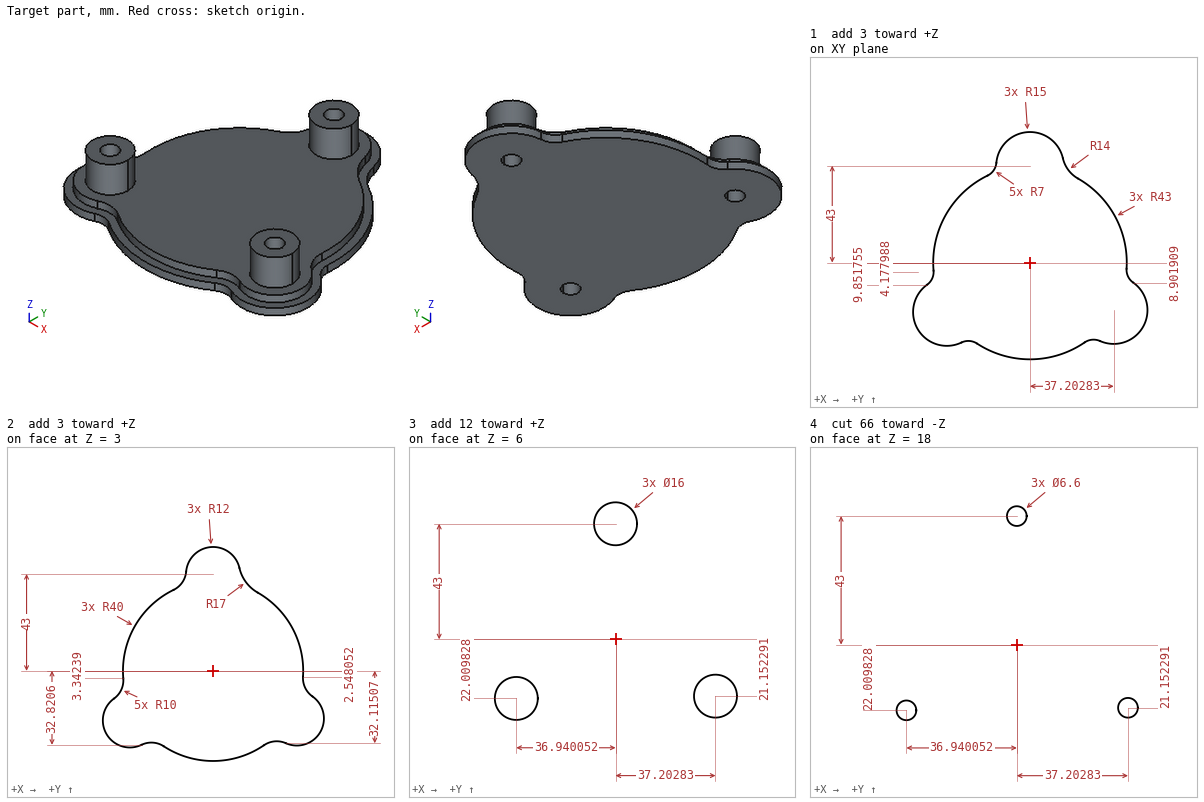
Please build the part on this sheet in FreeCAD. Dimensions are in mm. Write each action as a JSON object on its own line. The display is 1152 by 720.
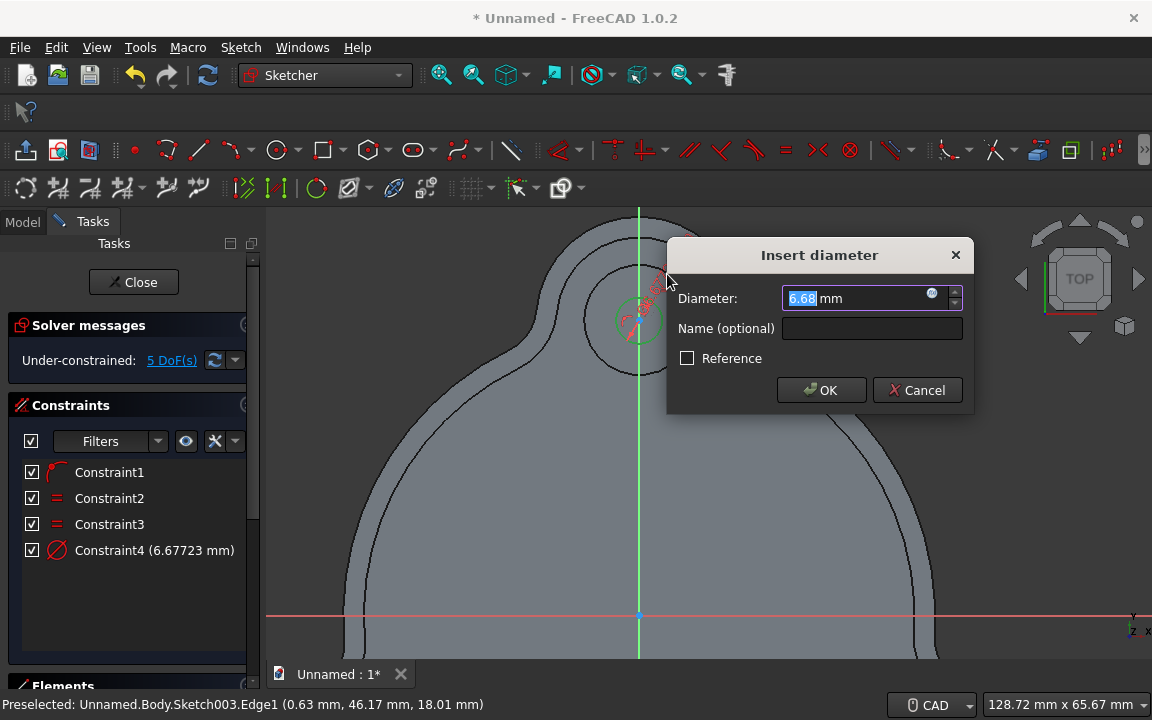
{"action": "type", "text": "6.6"}
{"action": "key", "text": "Return"}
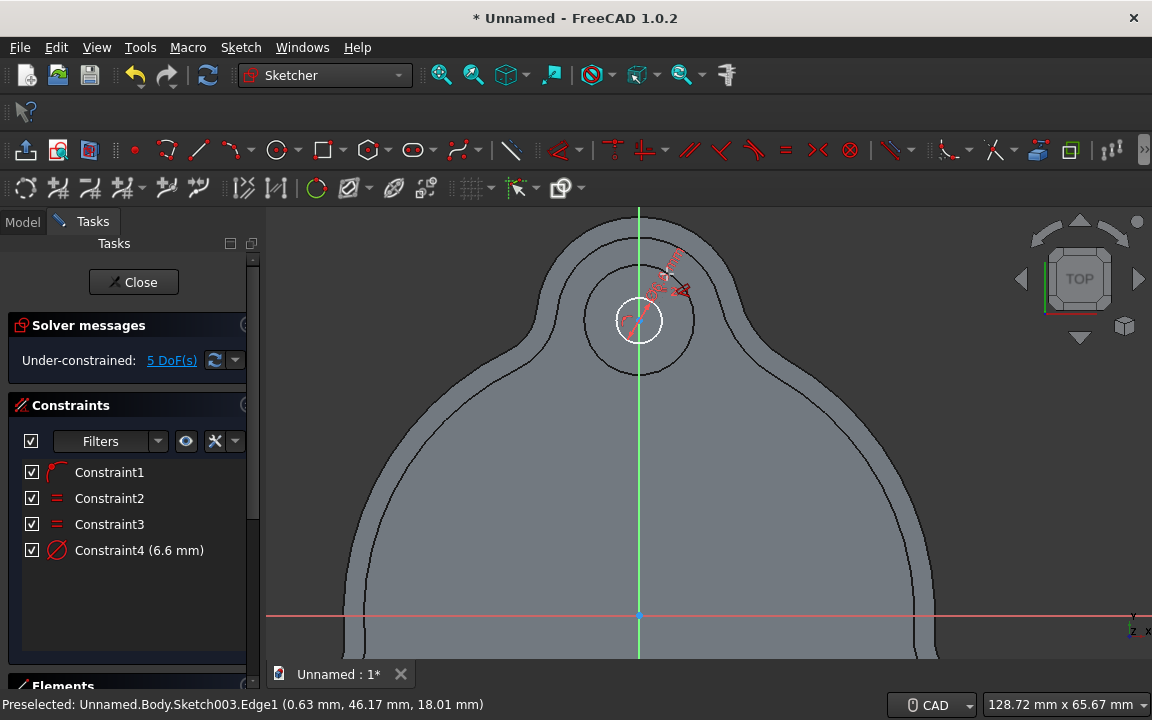
{"action": "left_click", "coordinate": [639, 321]}
{"action": "left_click", "coordinate": [605, 468]}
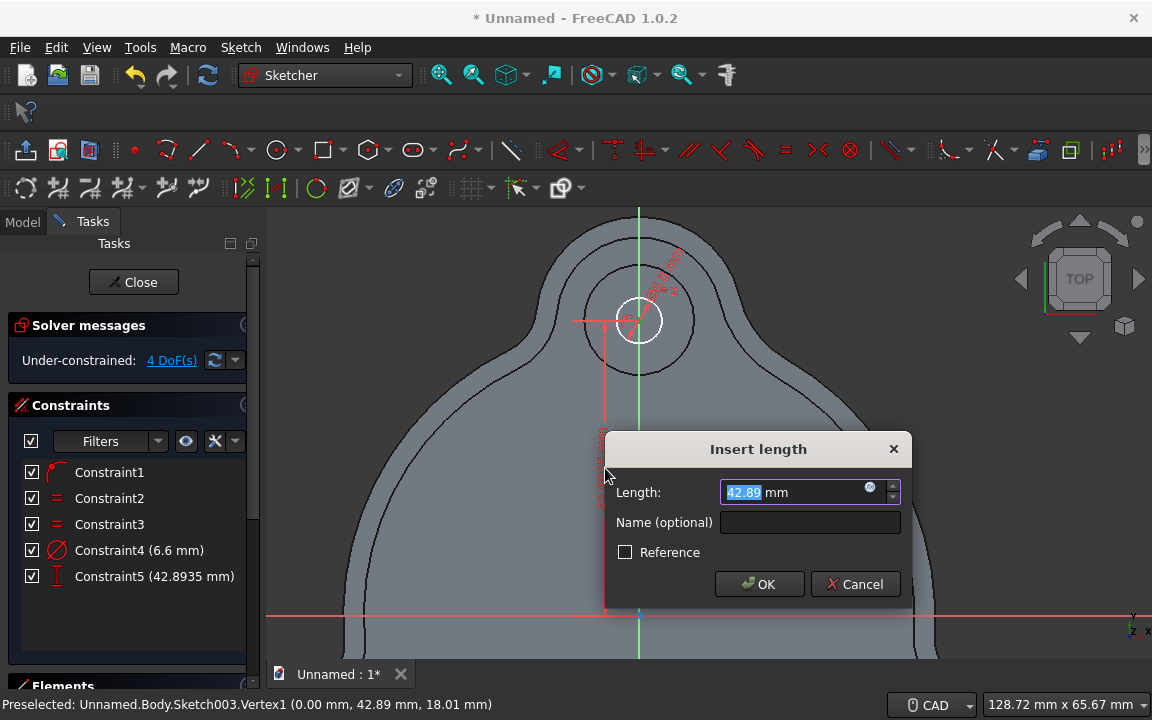
{"action": "type", "text": "43"}
{"action": "key", "text": "Return"}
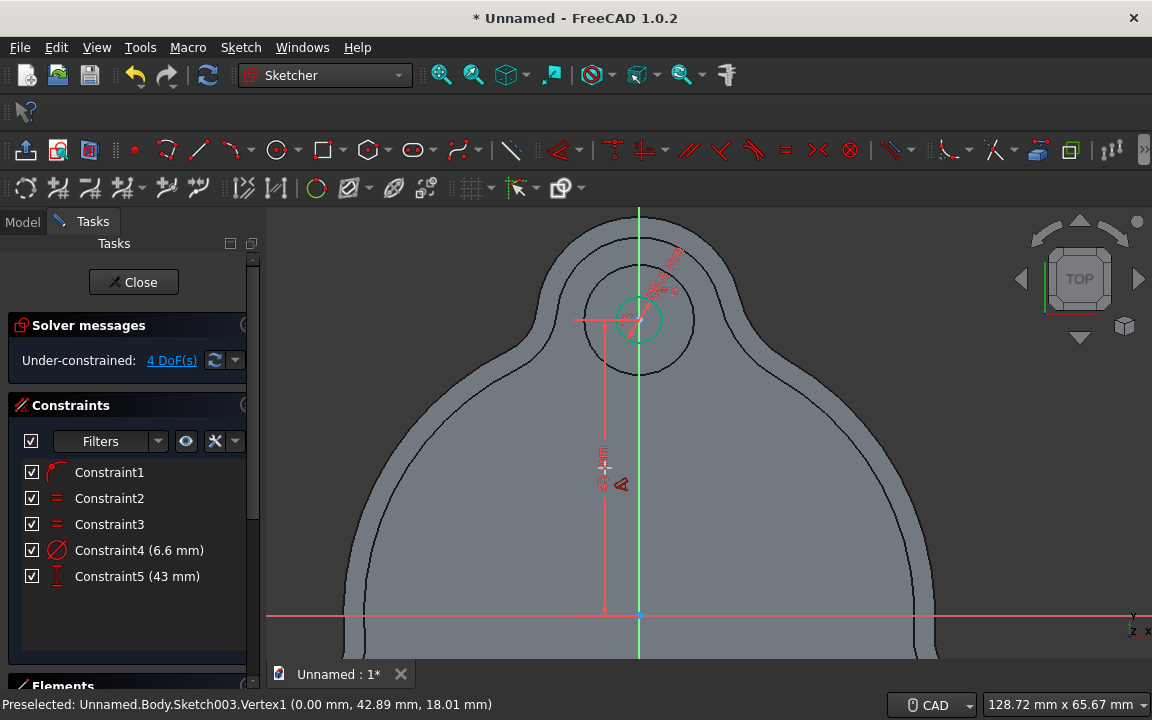
{"action": "scroll", "coordinate": [641, 298], "scroll_direction": "down", "scroll_amount": 3}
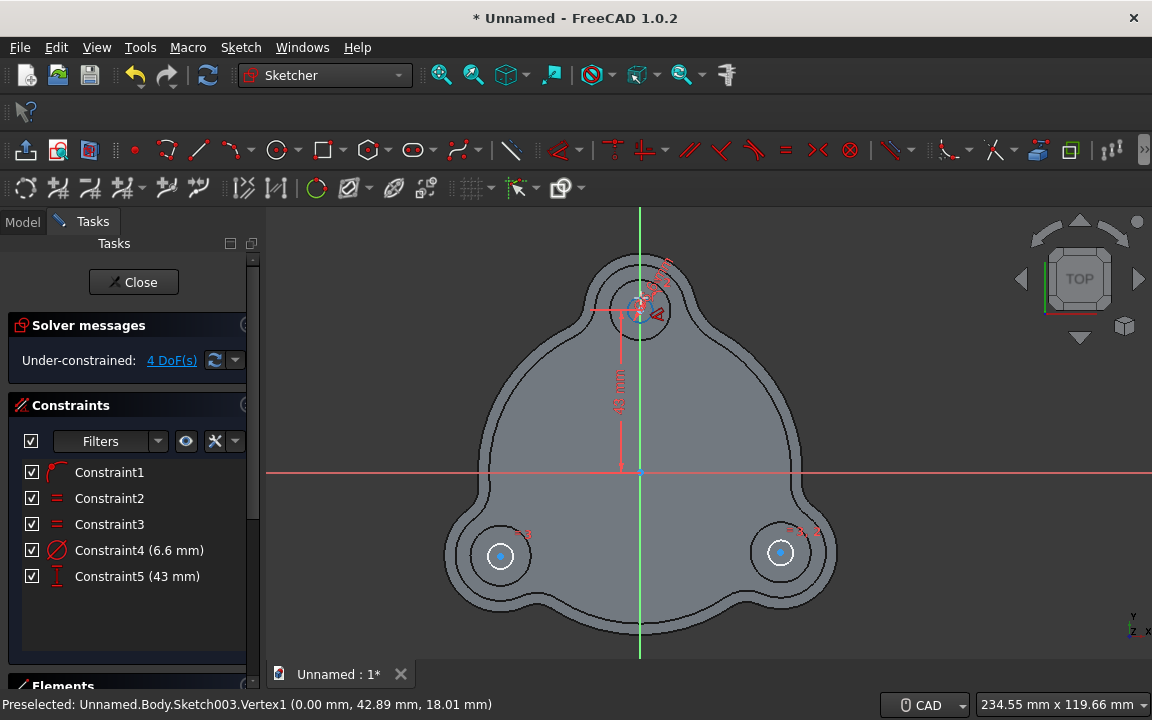
{"action": "left_click", "coordinate": [781, 553]}
{"action": "left_click", "coordinate": [710, 587]}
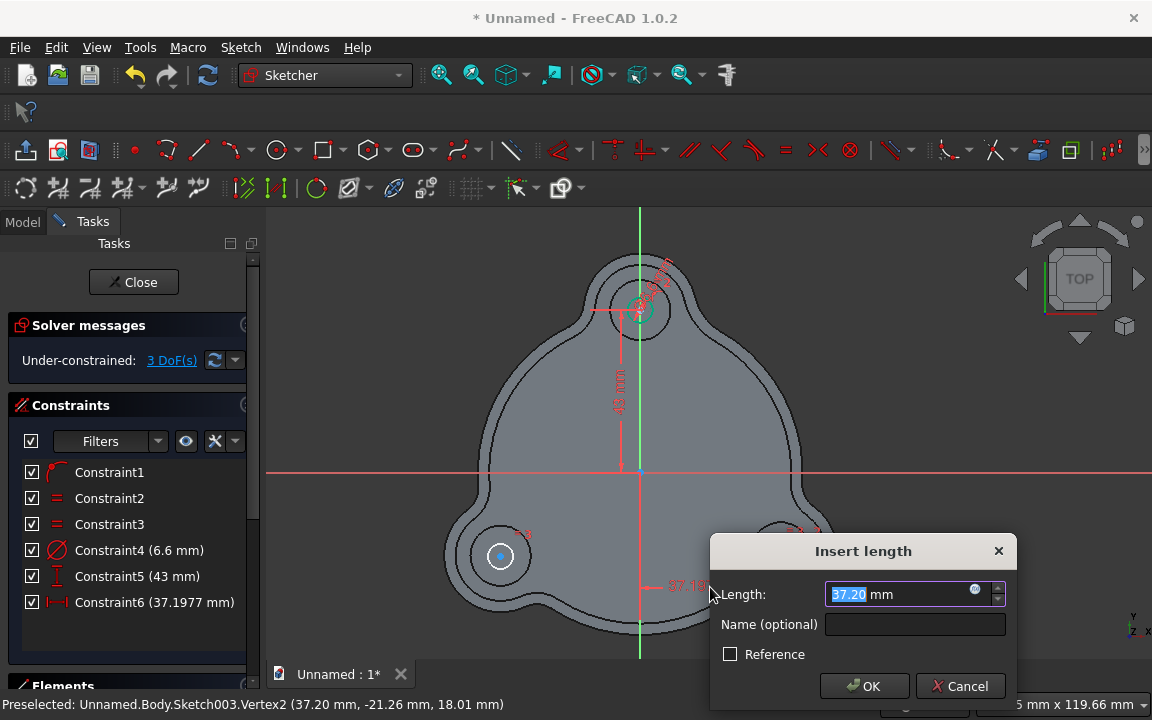
{"action": "type", "text": "37.20283"}
{"action": "key", "text": "Return"}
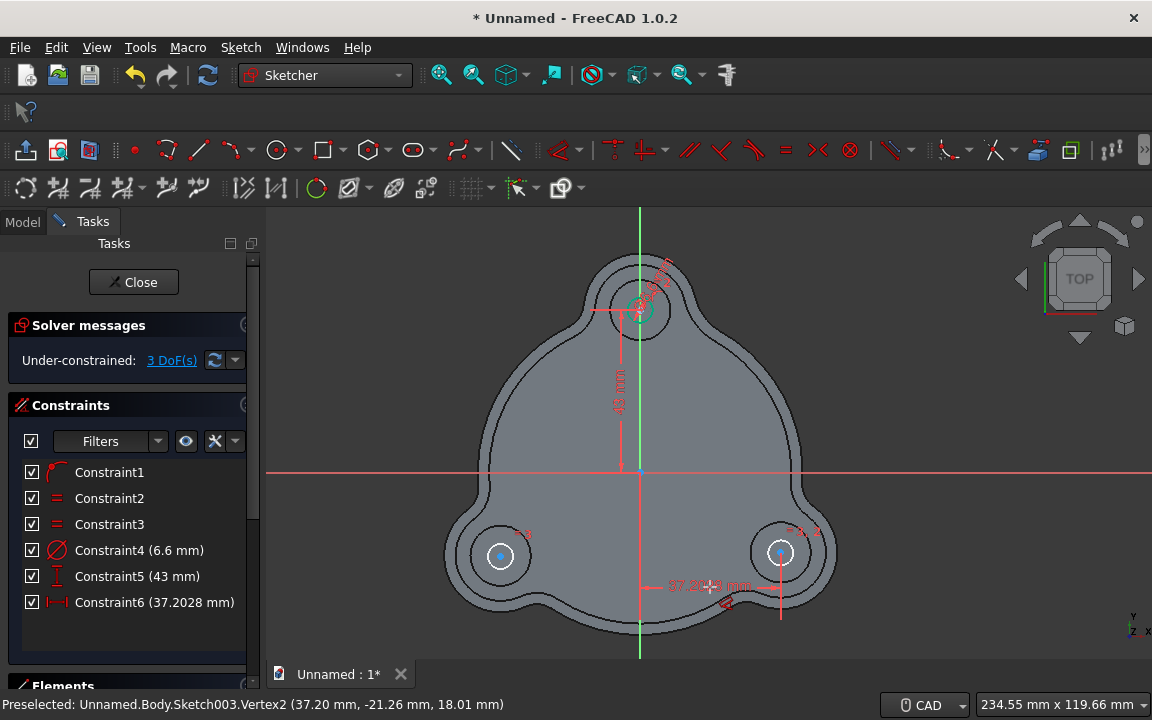
{"action": "left_click", "coordinate": [781, 553]}
{"action": "left_click", "coordinate": [815, 513]}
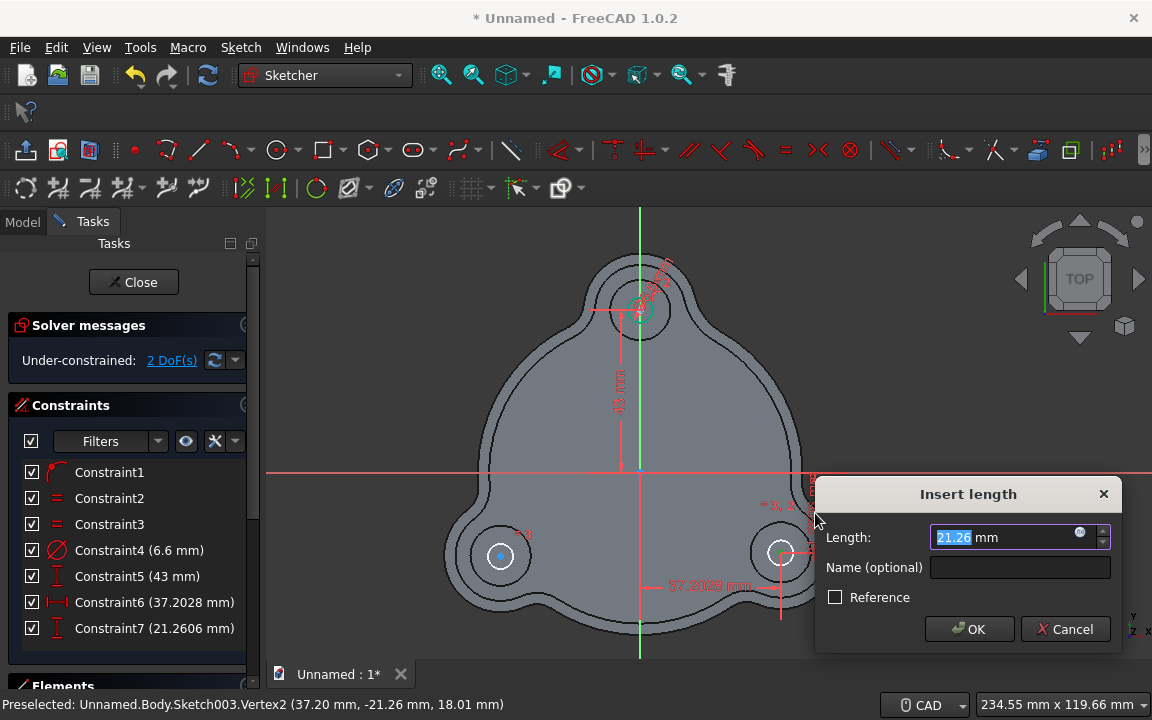
{"action": "type", "text": "21.152291"}
{"action": "key", "text": "Return"}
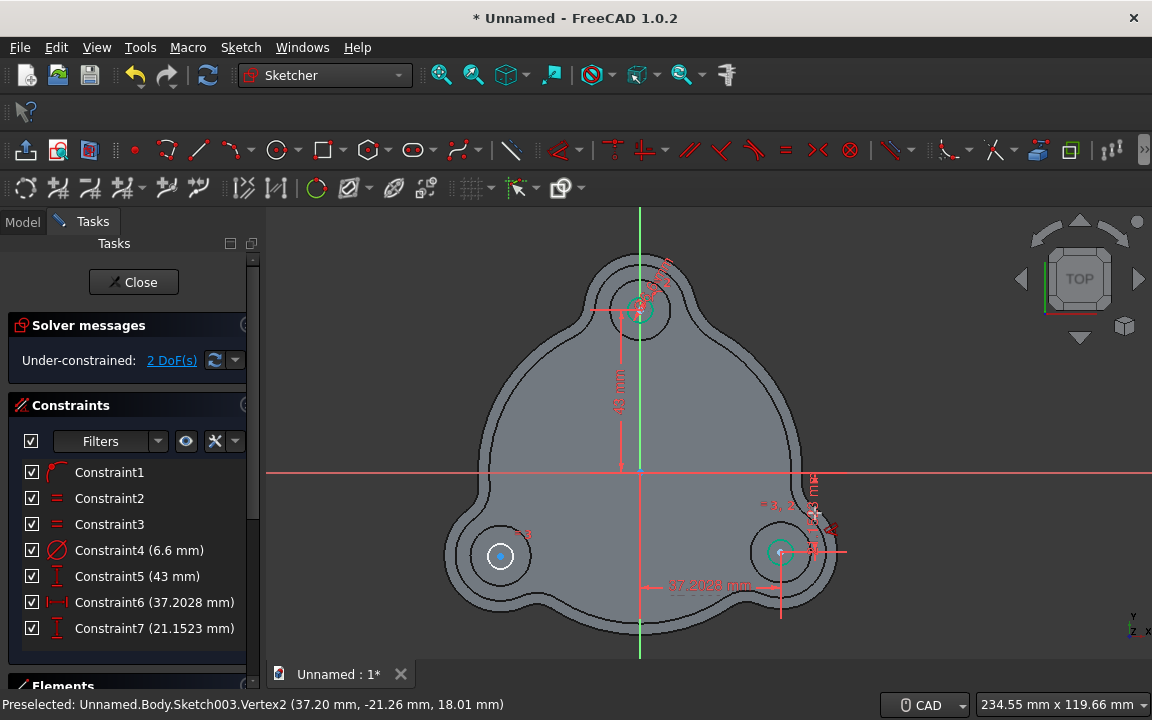
{"action": "left_click", "coordinate": [501, 556]}
{"action": "left_click", "coordinate": [570, 590]}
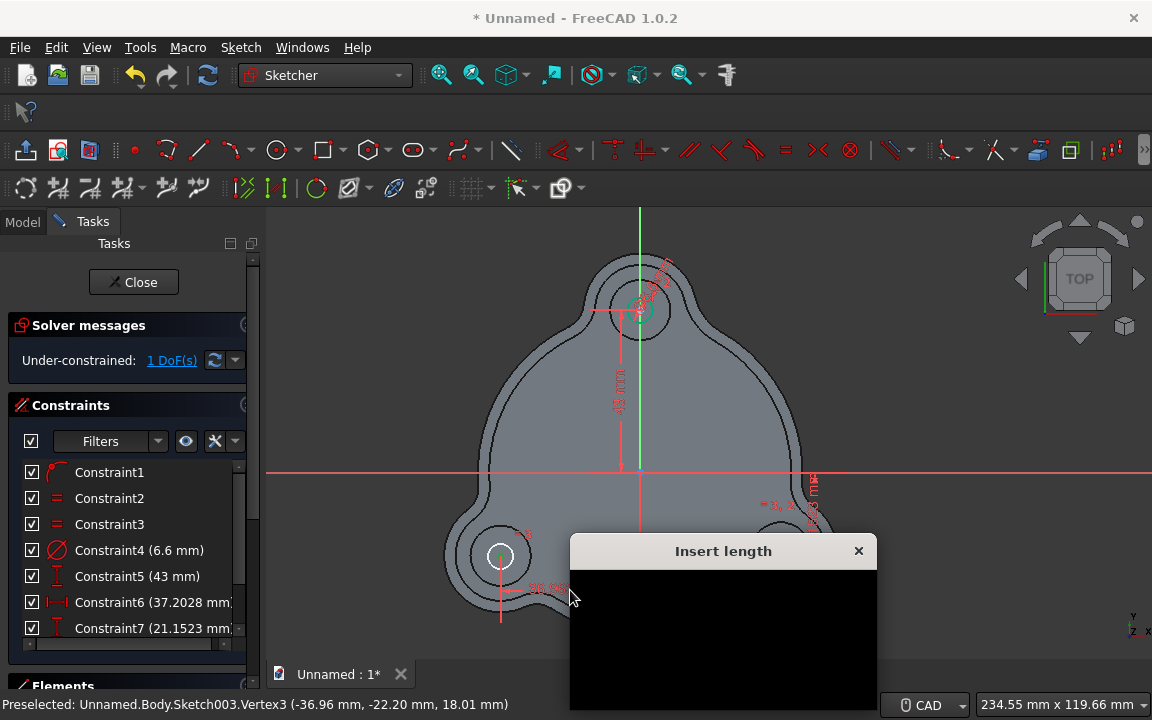
{"action": "type", "text": "36.940052"}
{"action": "key", "text": "Return"}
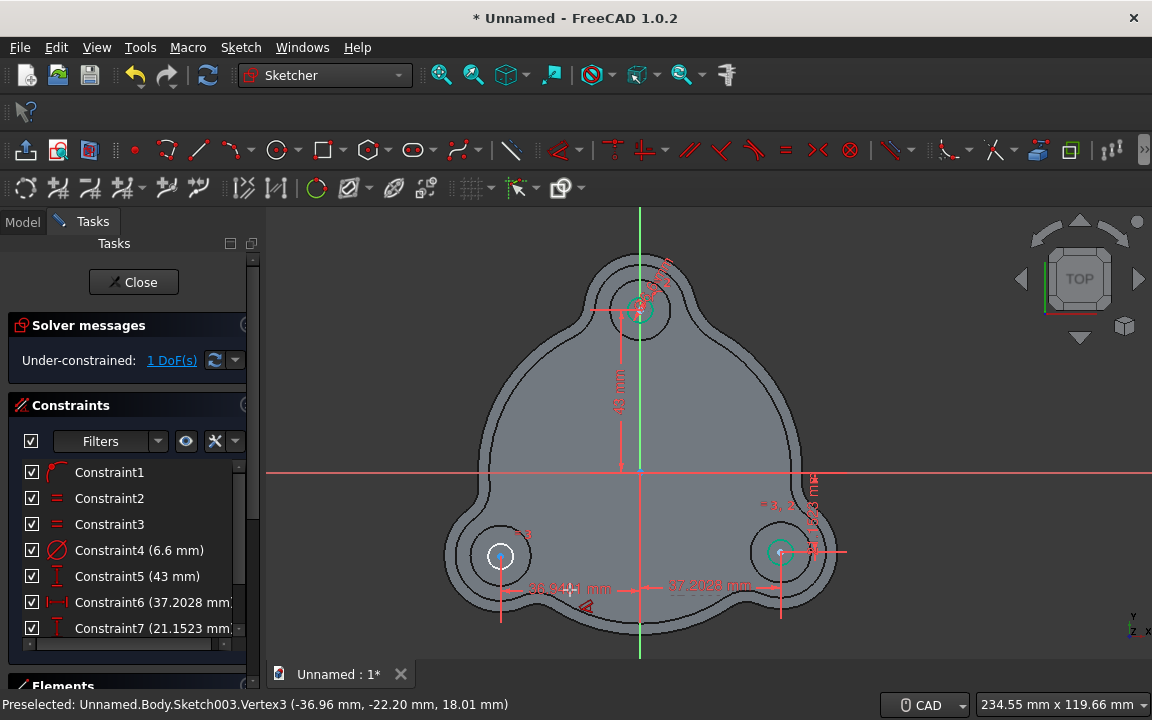
{"action": "left_click", "coordinate": [501, 556]}
{"action": "left_click", "coordinate": [467, 515]}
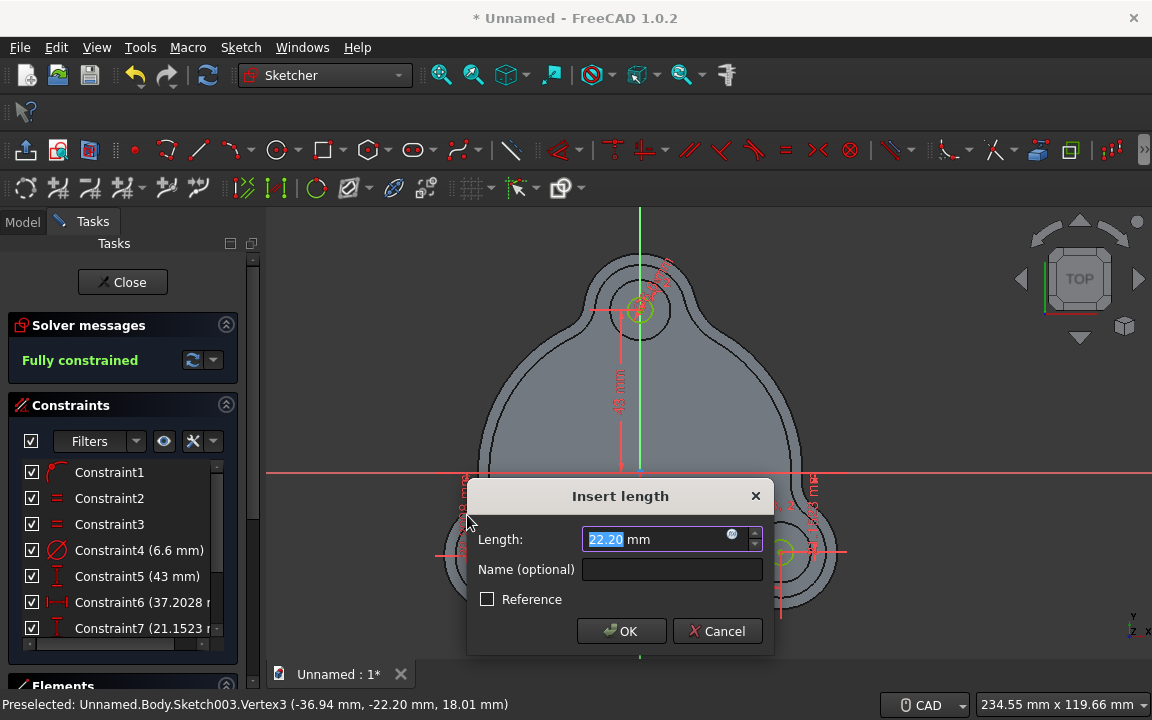
{"action": "type", "text": "22.009828"}
{"action": "key", "text": "Return"}
{"action": "key", "text": "Escape"}